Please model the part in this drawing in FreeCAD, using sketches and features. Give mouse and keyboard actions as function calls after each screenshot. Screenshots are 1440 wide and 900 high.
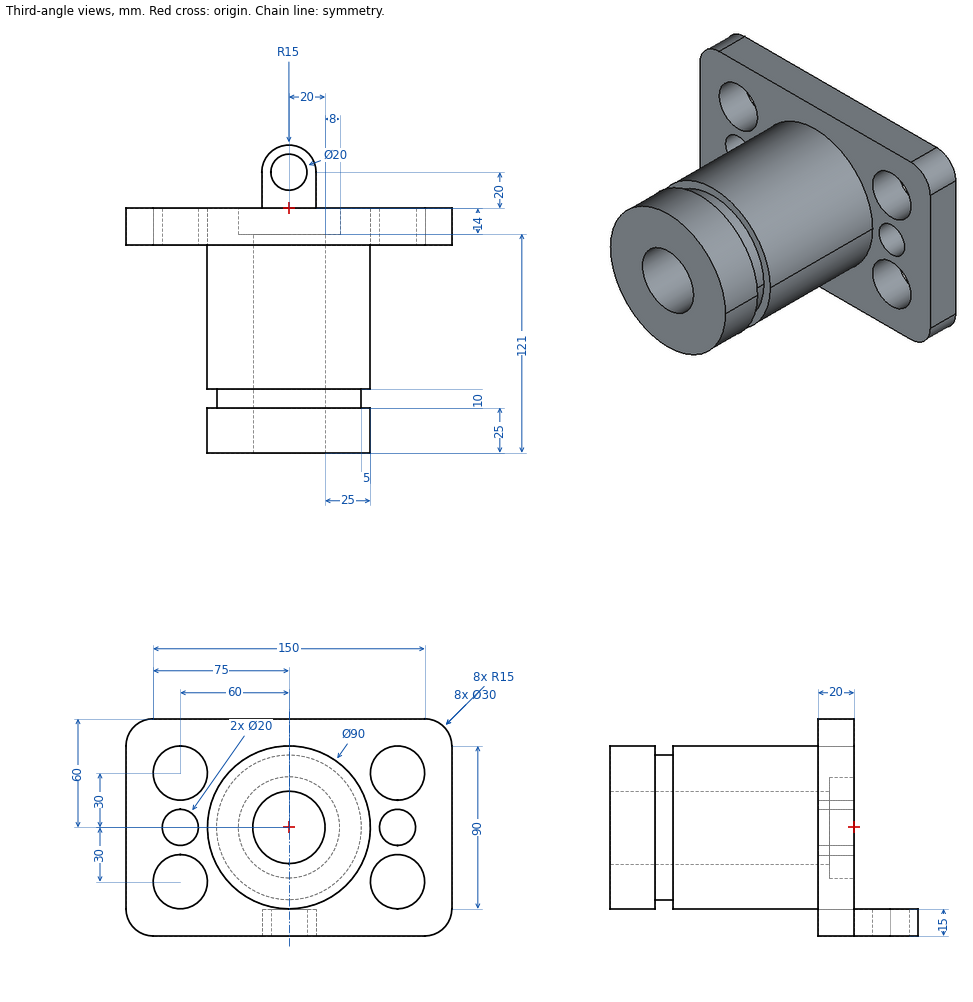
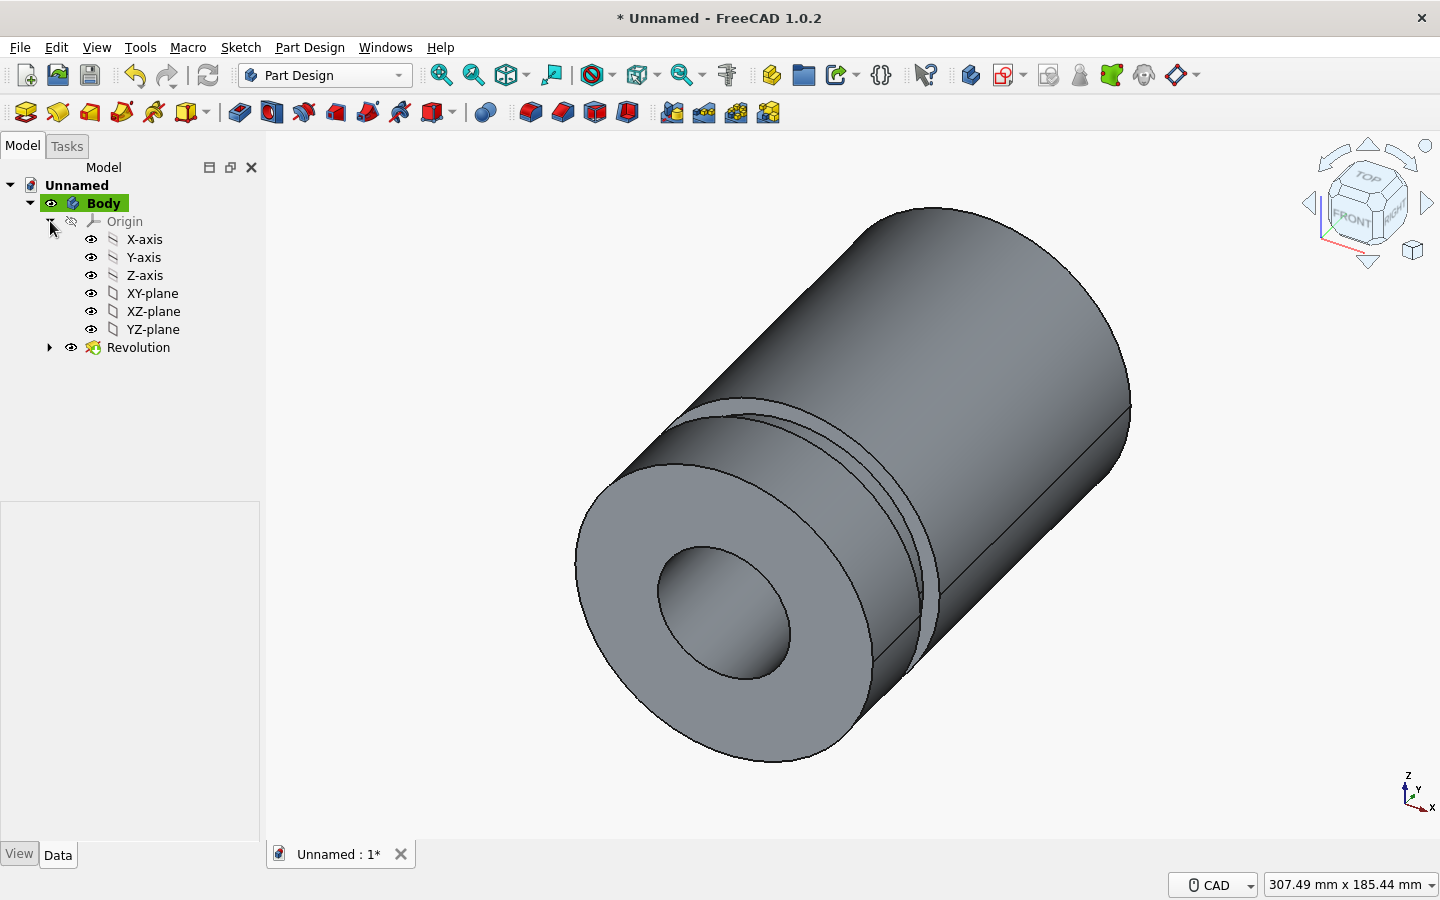
click(136, 311)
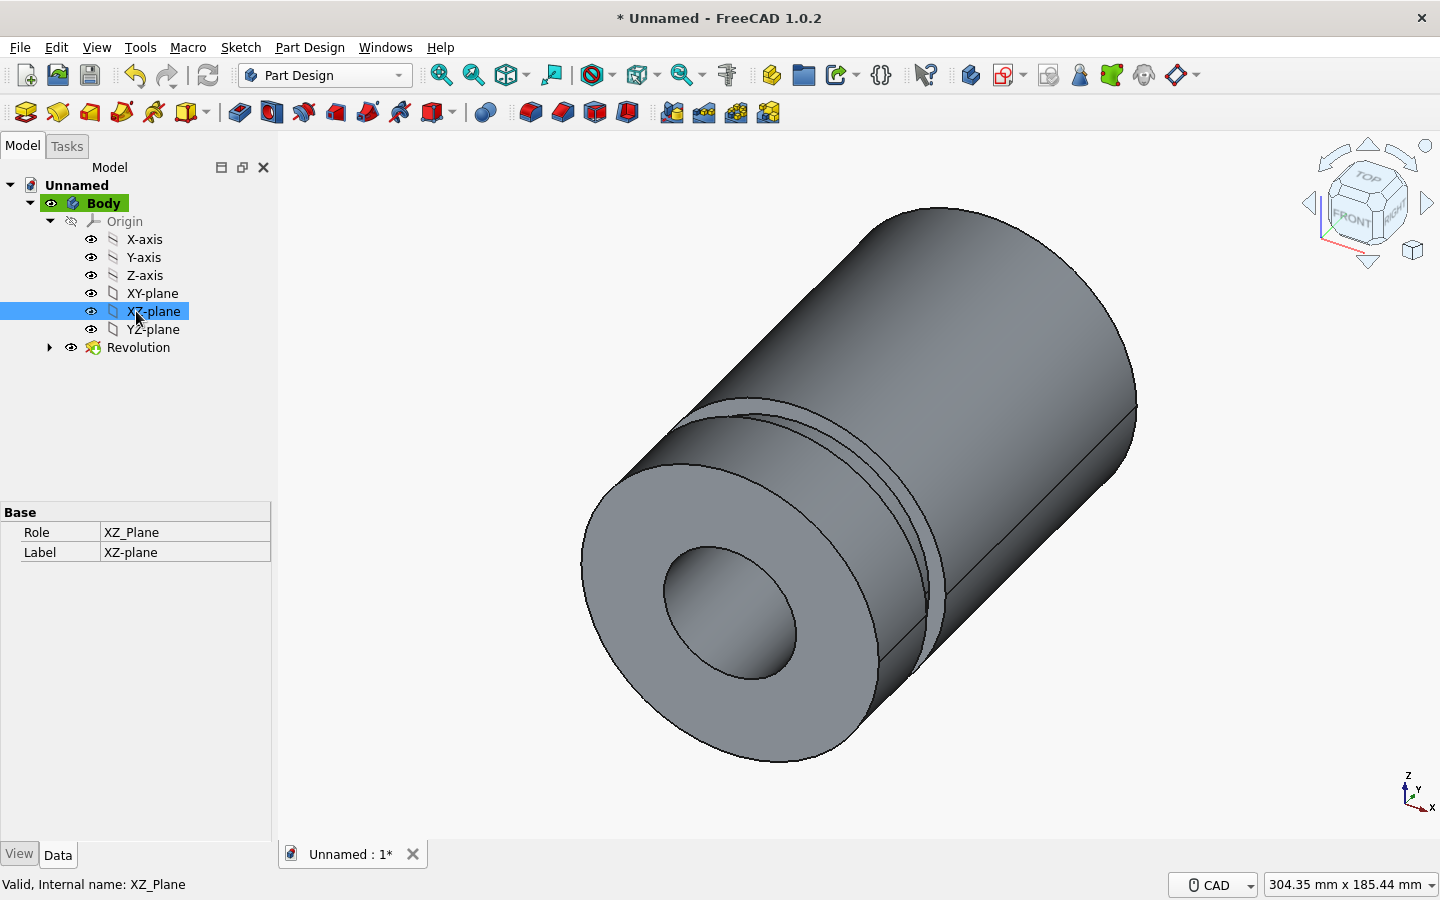
click(1176, 76)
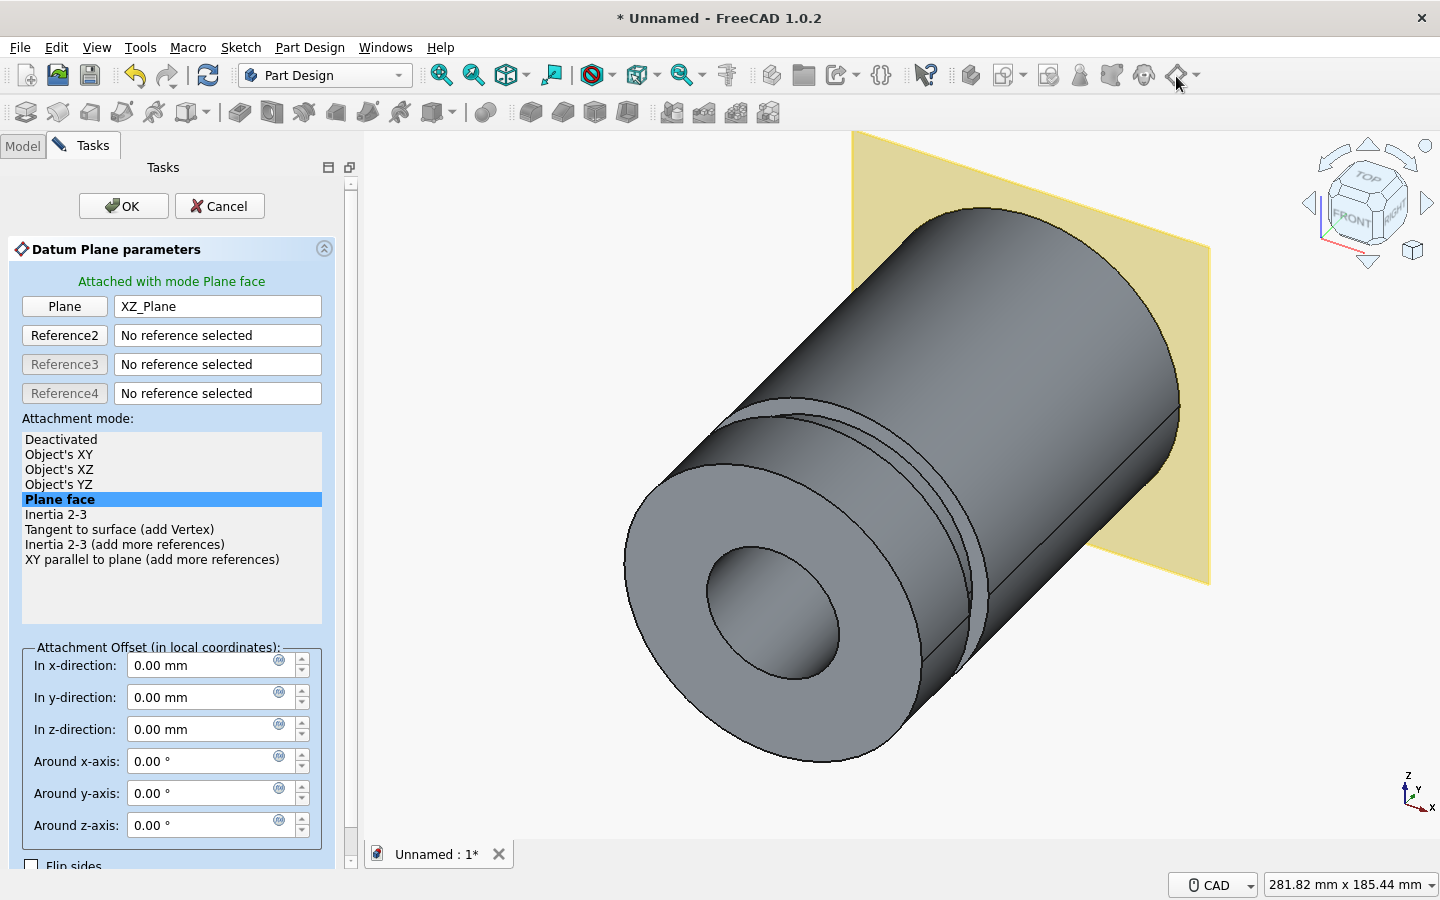
triple_click(210, 729)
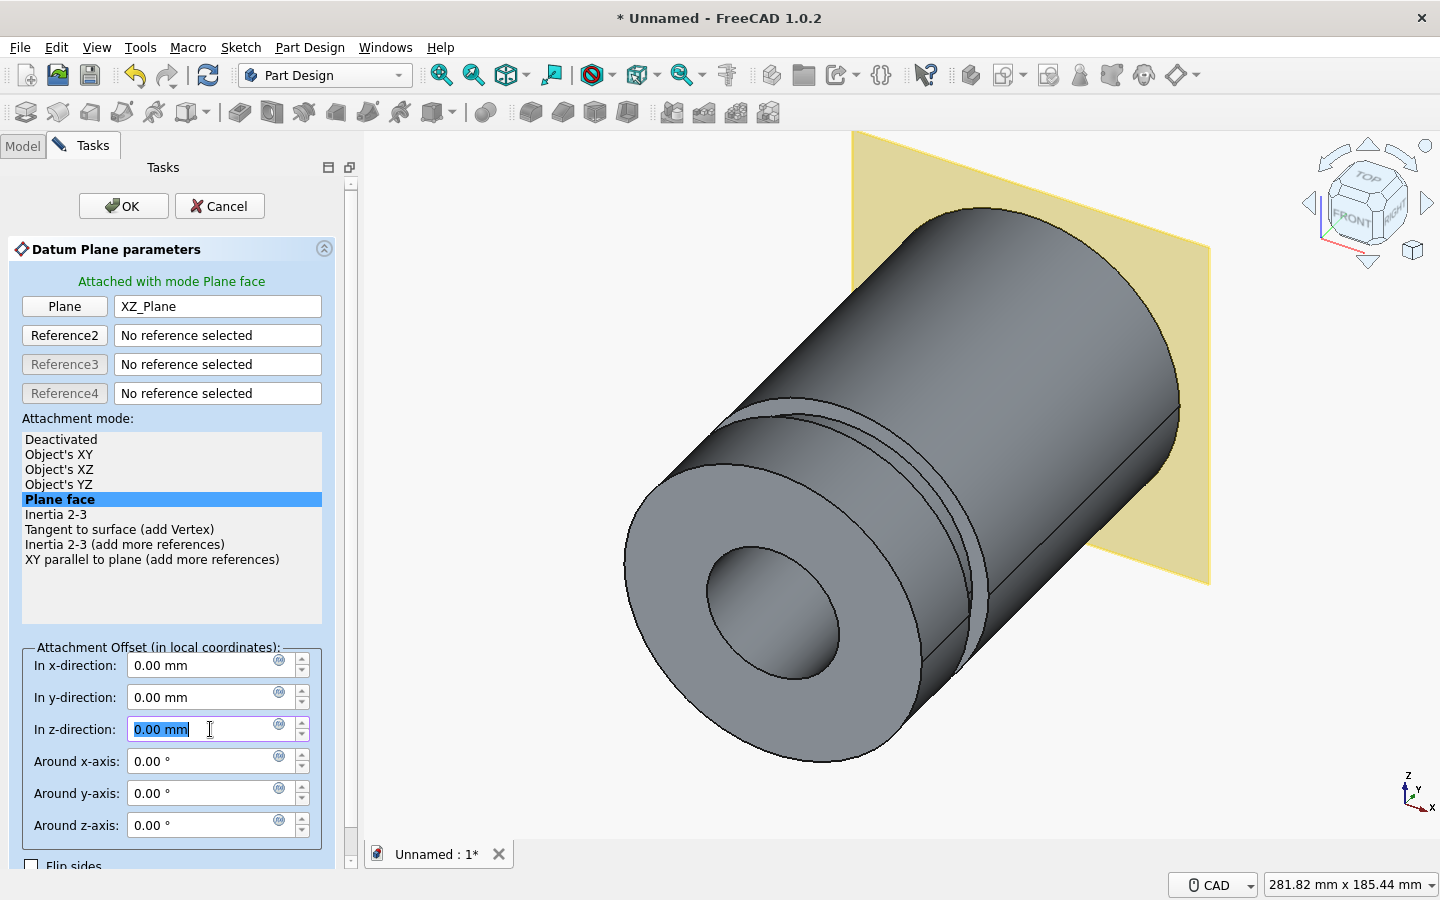
text(20)
key(Tab)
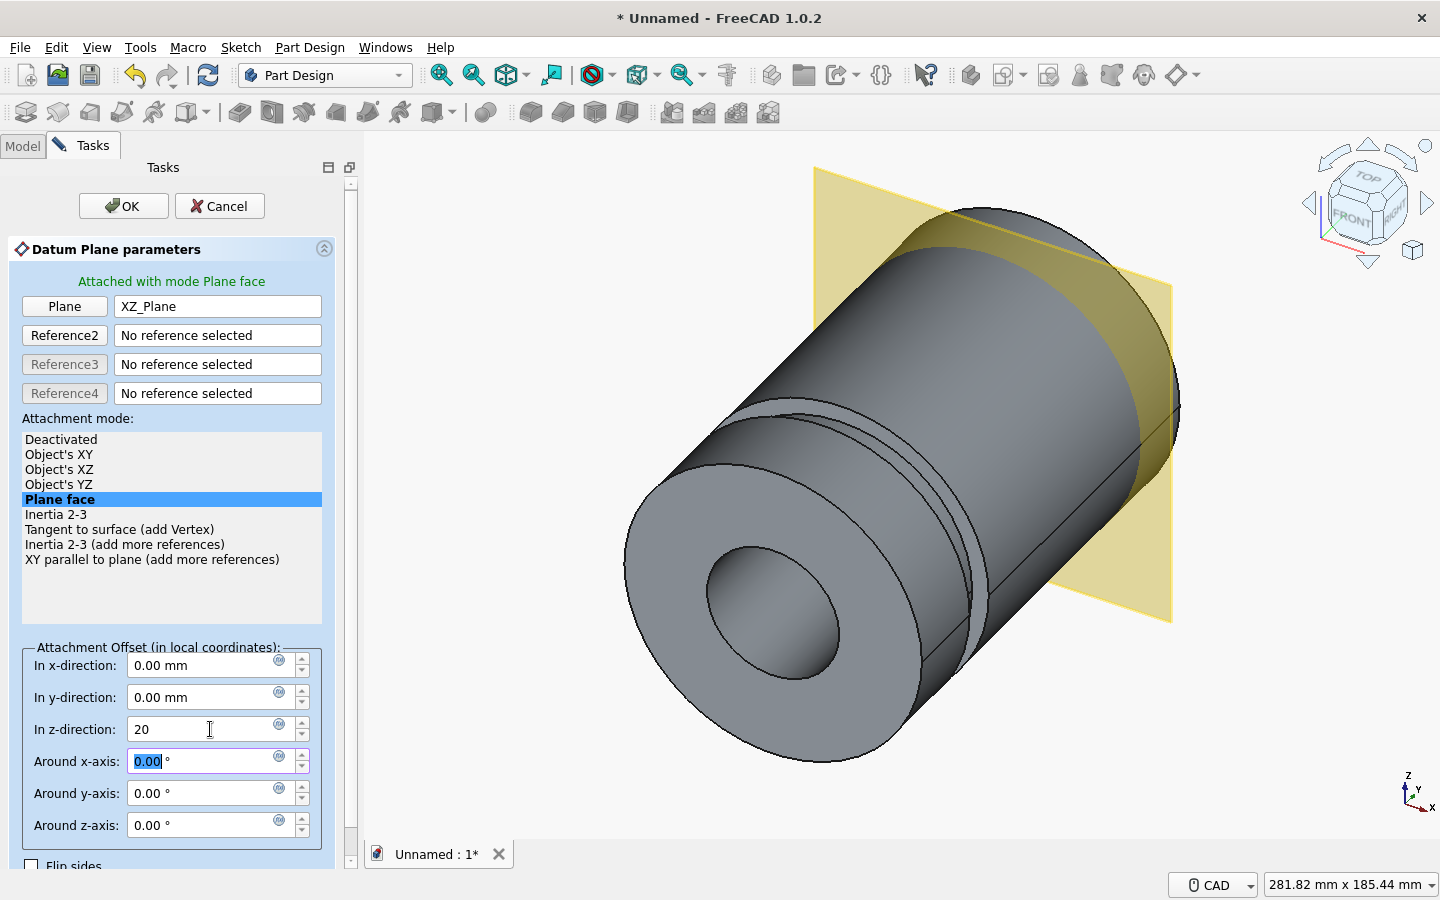
click(124, 206)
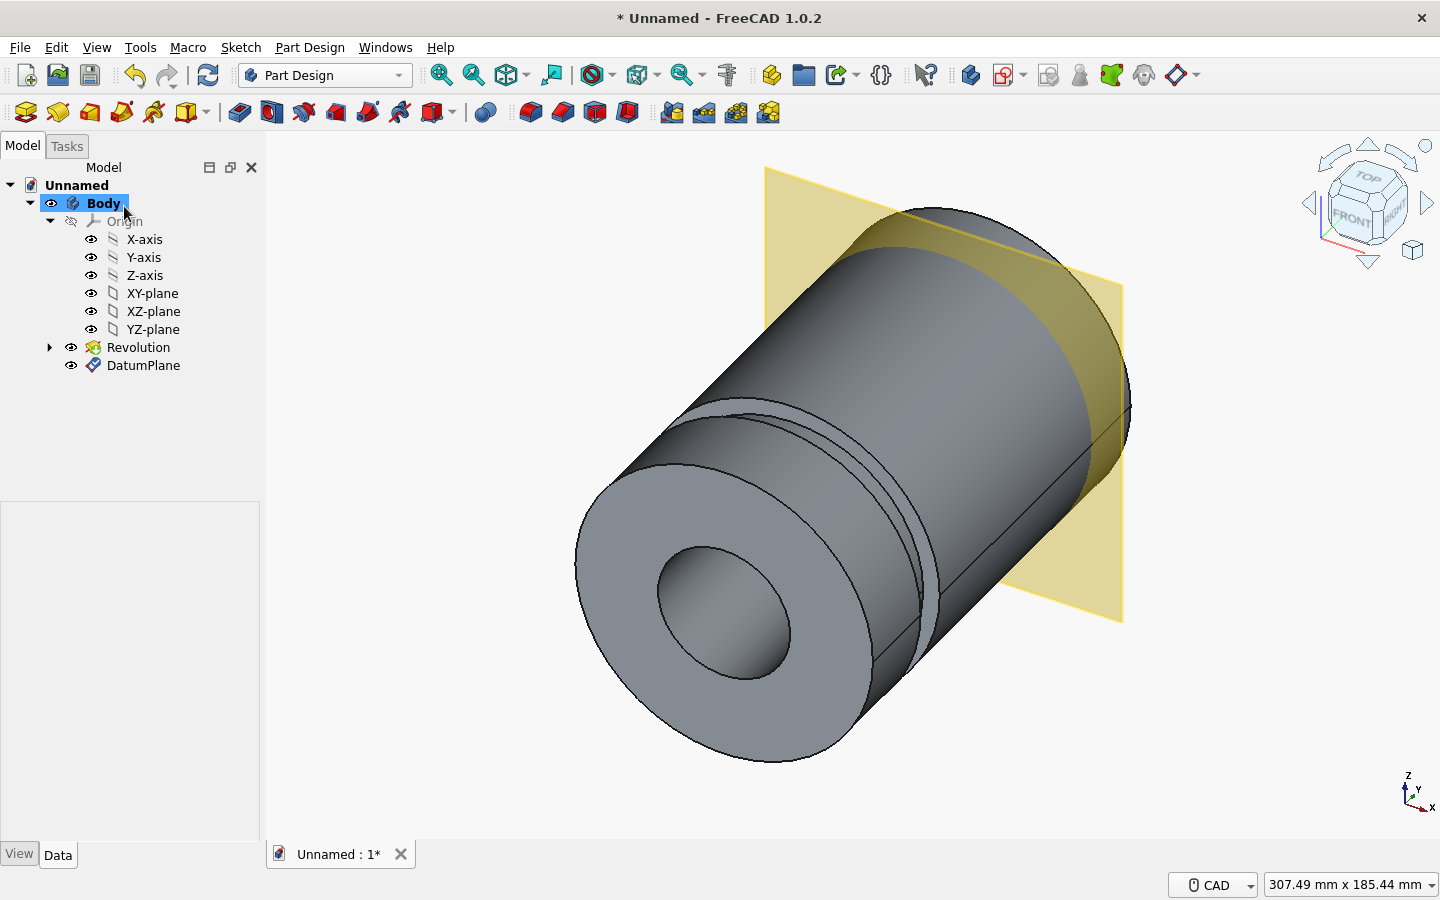
click(116, 365)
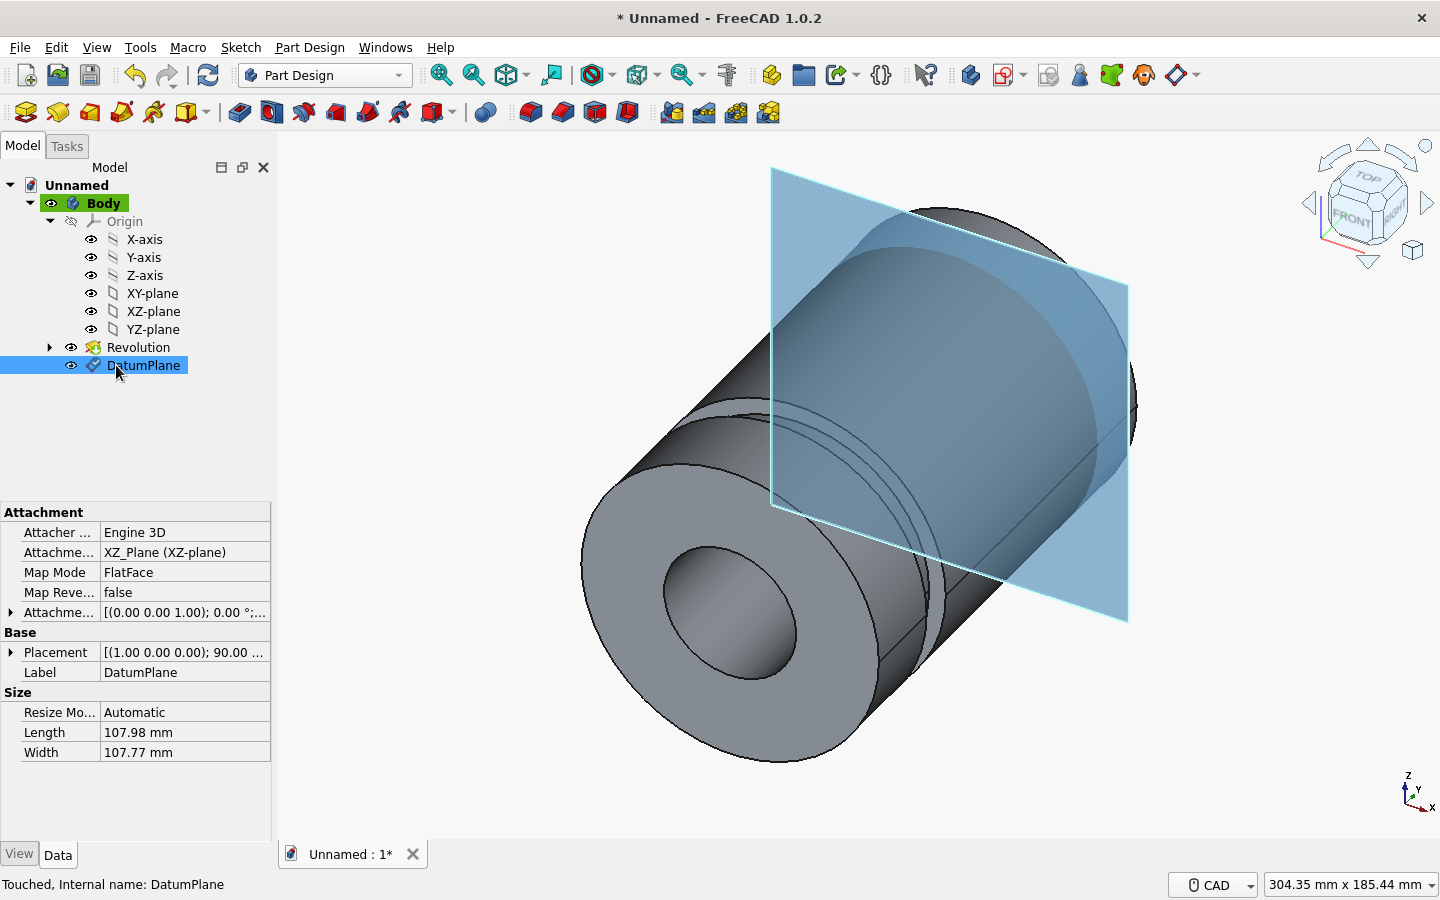
click(1004, 76)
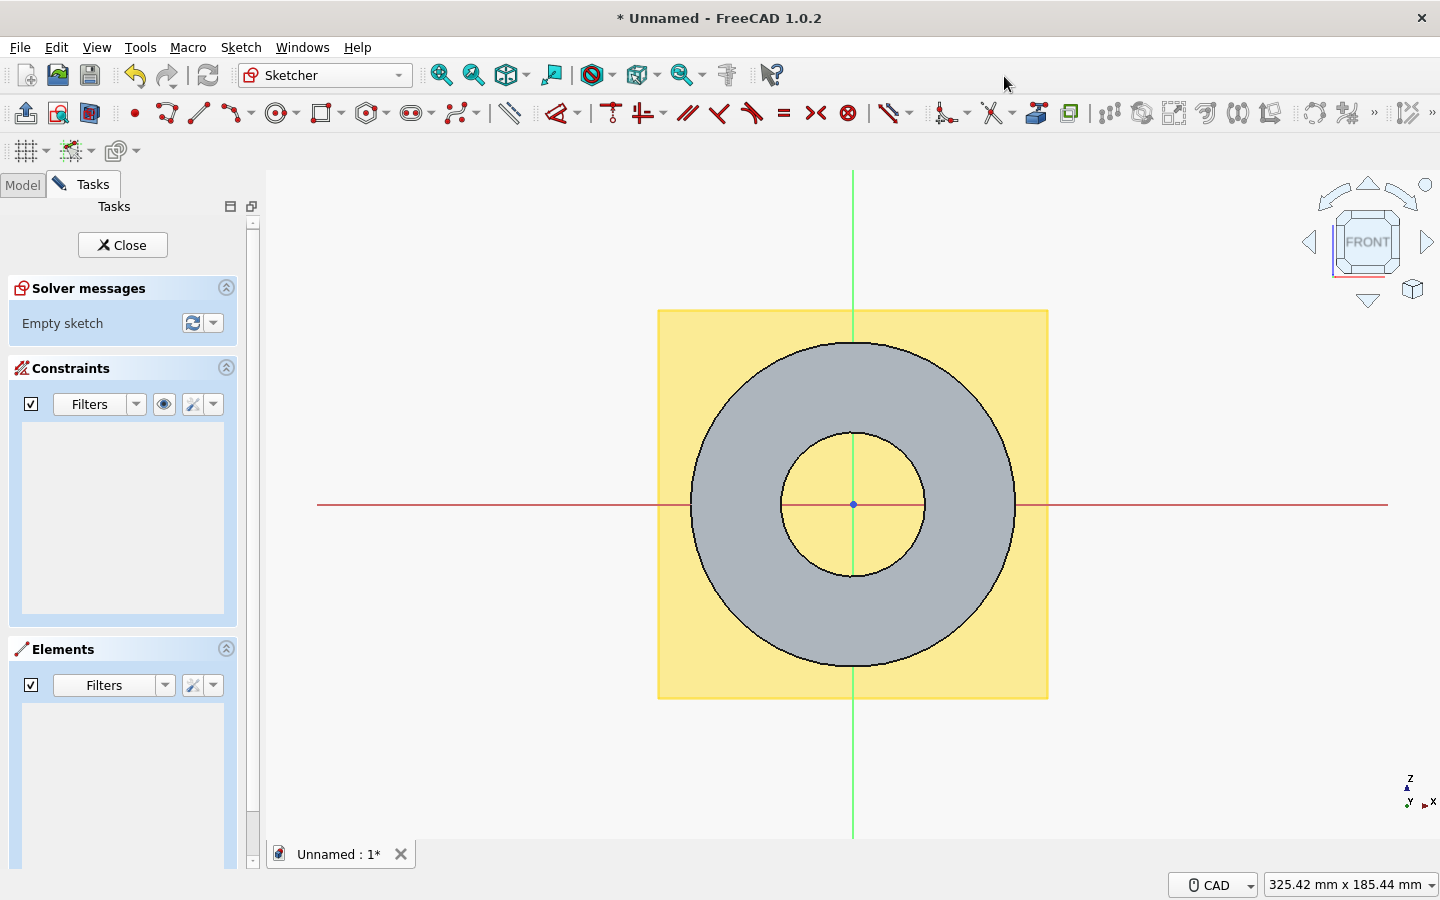
key(q)
key(s)